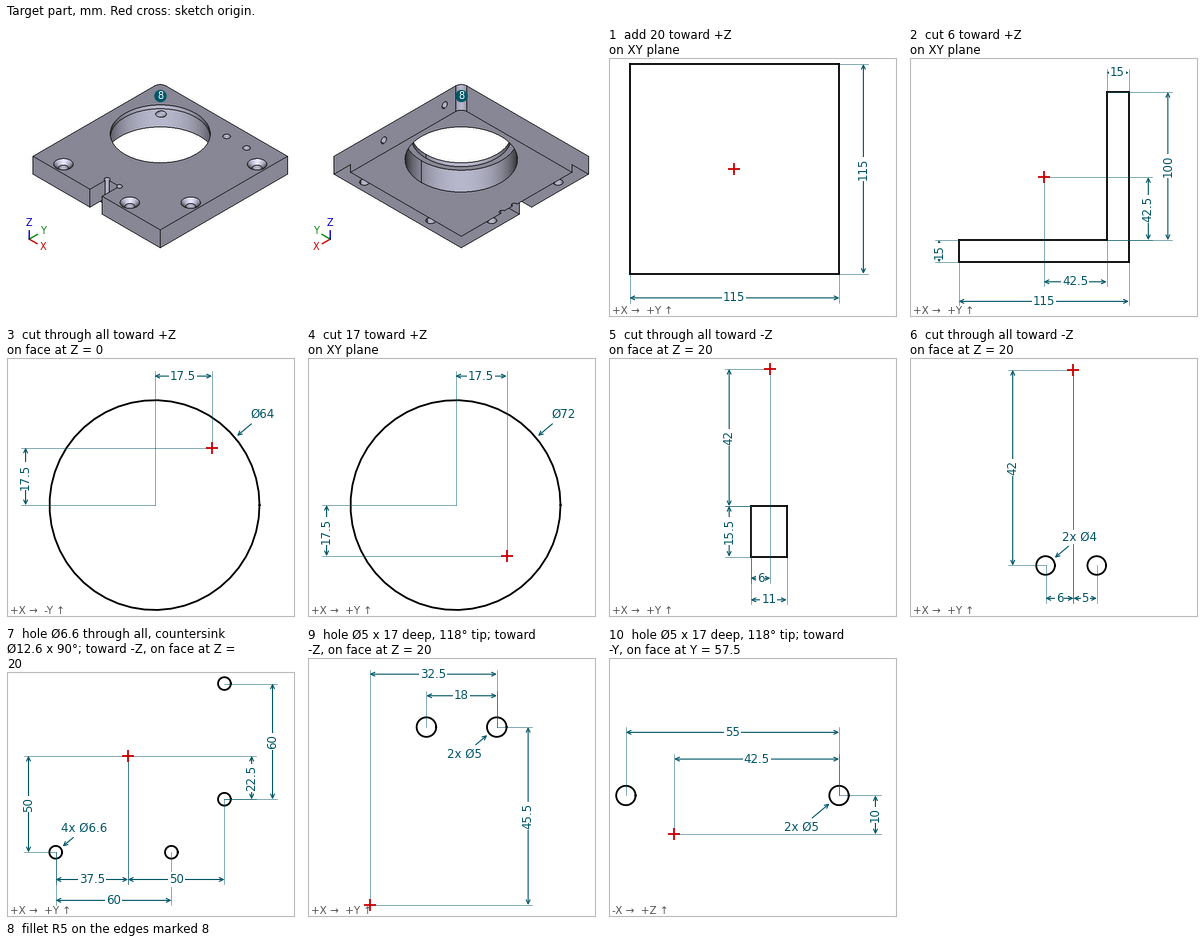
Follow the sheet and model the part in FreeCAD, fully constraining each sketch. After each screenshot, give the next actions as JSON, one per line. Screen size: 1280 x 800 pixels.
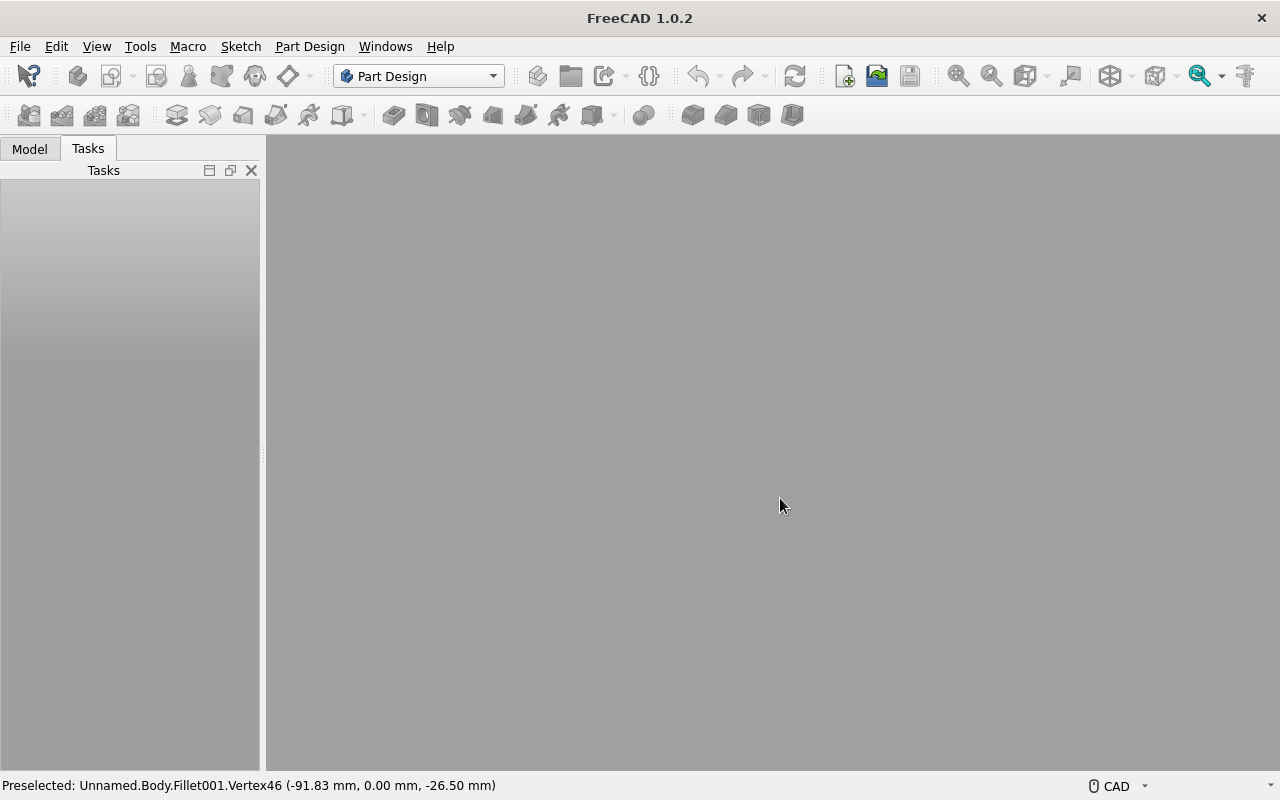
{"action": "key", "text": "ctrl+n"}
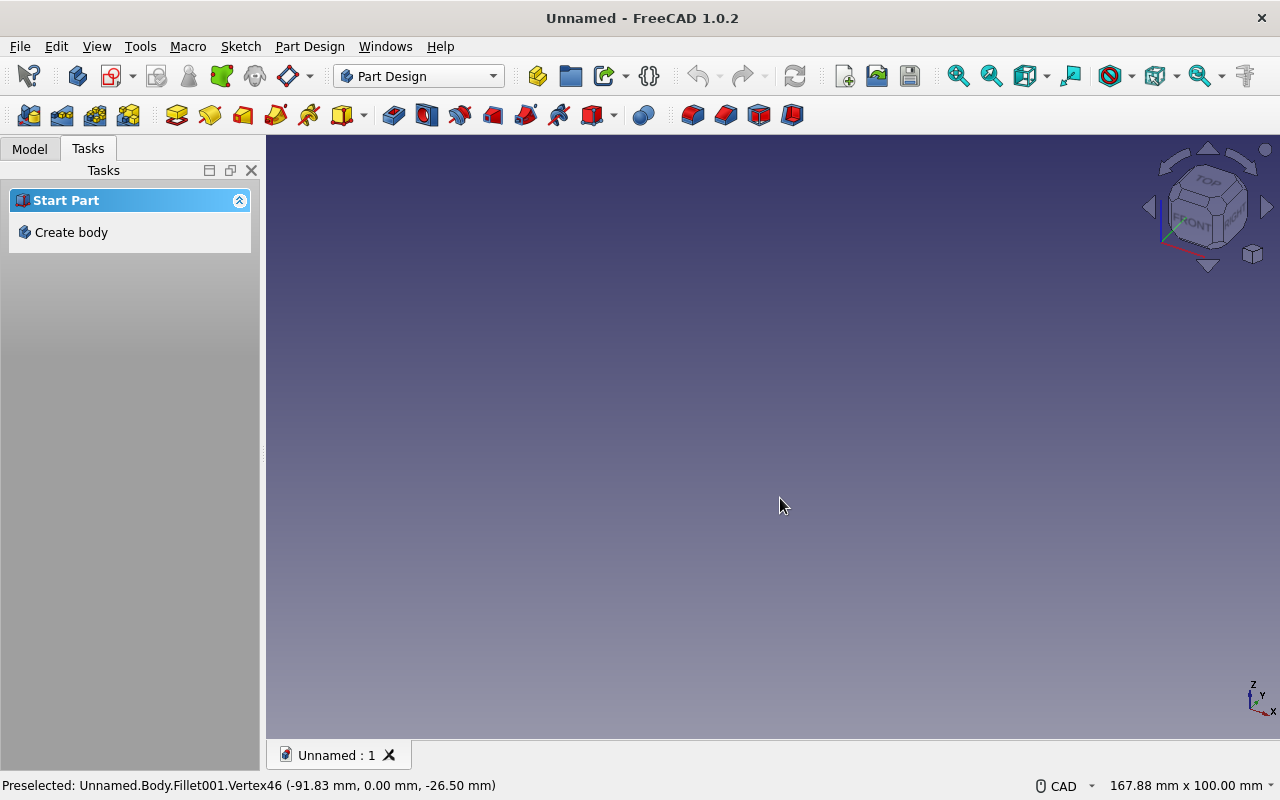
{"action": "left_click", "coordinate": [110, 76]}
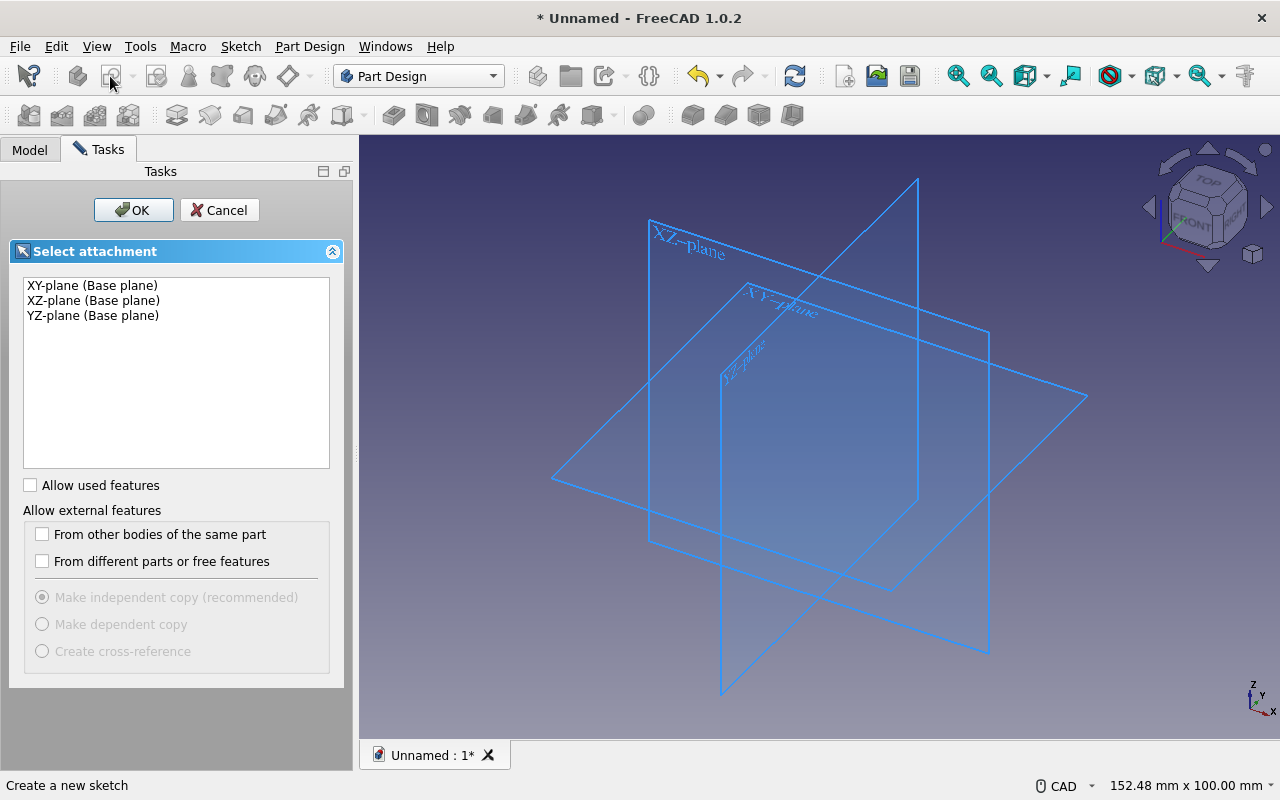
{"action": "left_click", "coordinate": [84, 286]}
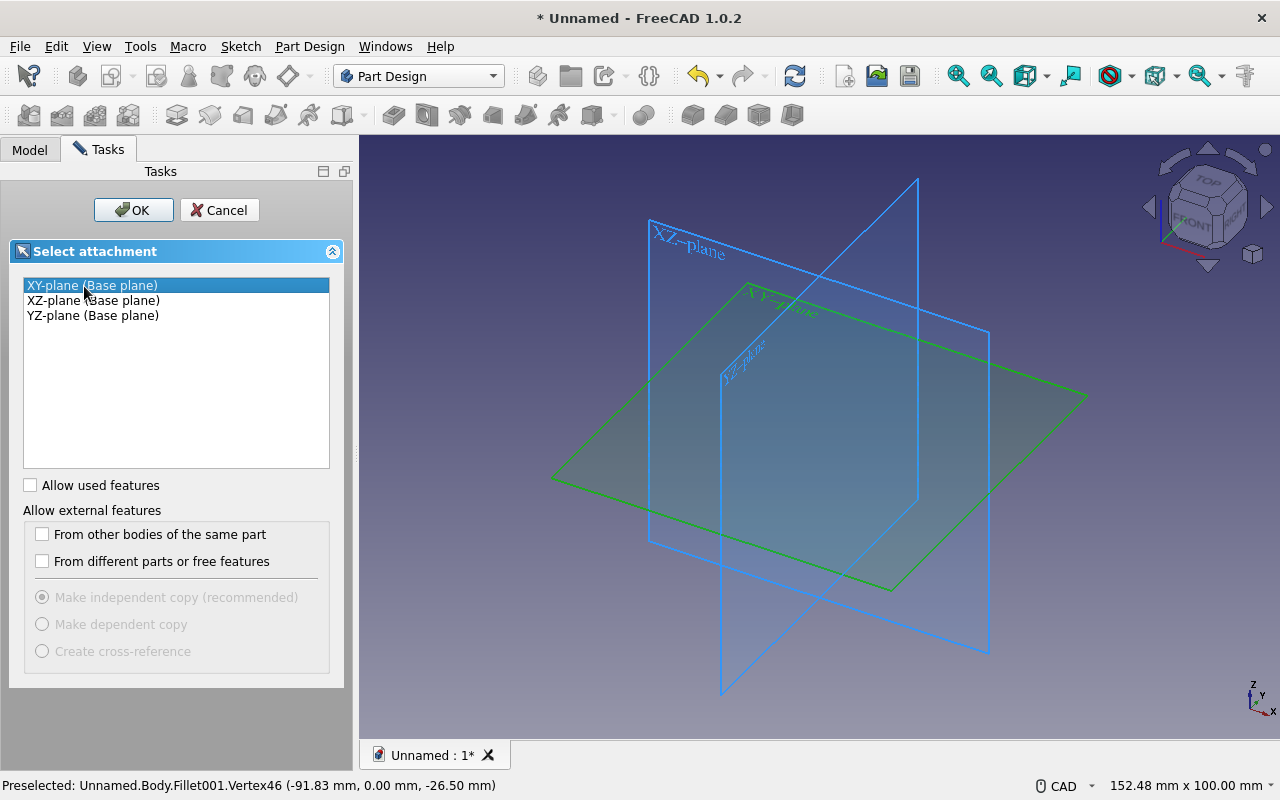
{"action": "left_click", "coordinate": [134, 210]}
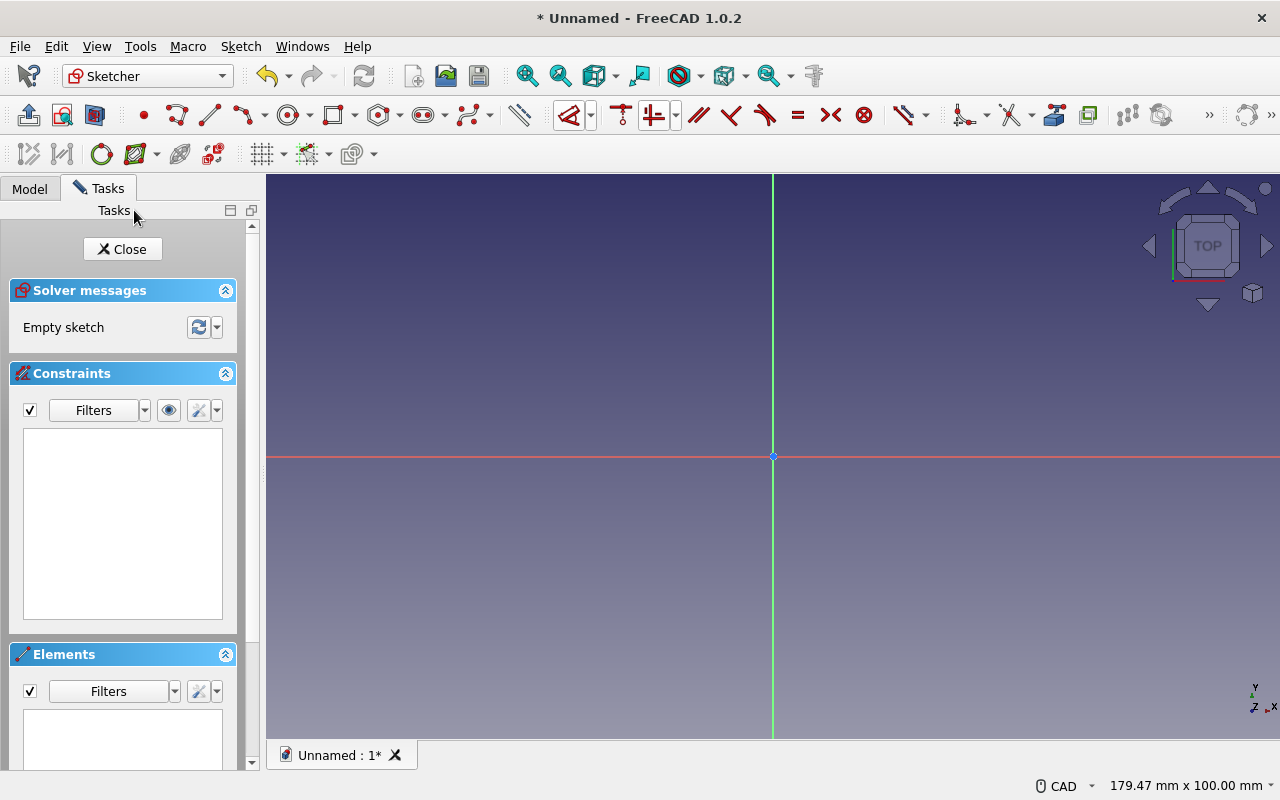
{"action": "scroll", "coordinate": [621, 456], "scroll_direction": "down", "scroll_amount": 3}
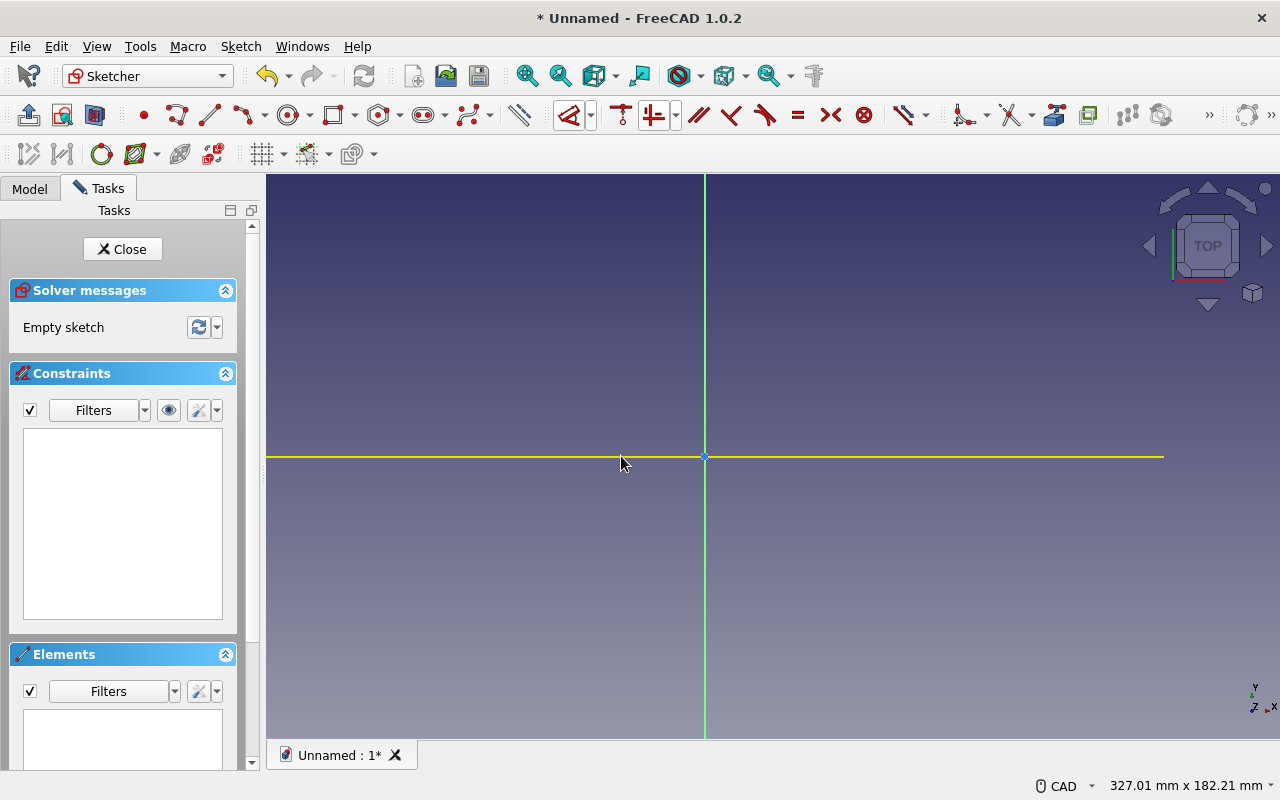
{"action": "key", "text": "g v"}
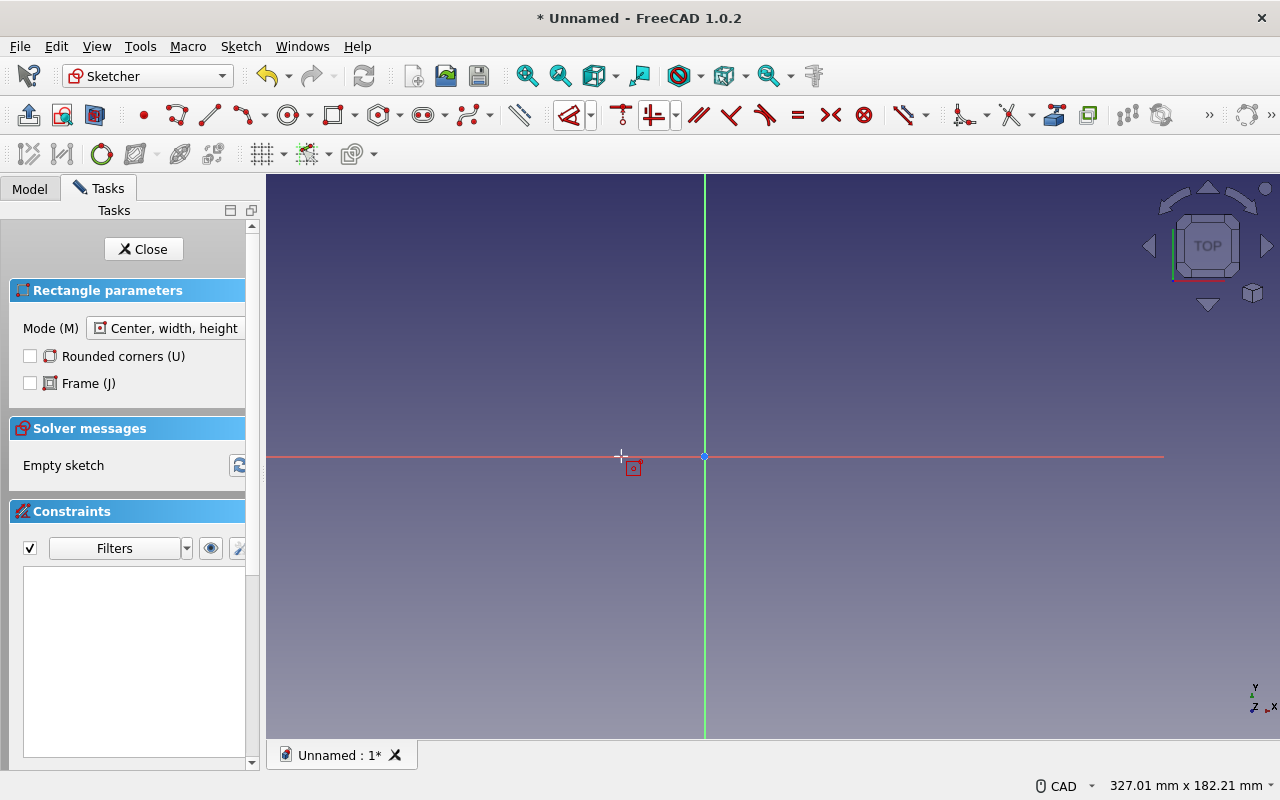
{"action": "left_click", "coordinate": [705, 456]}
{"action": "left_click", "coordinate": [883, 278]}
{"action": "key", "text": "Escape"}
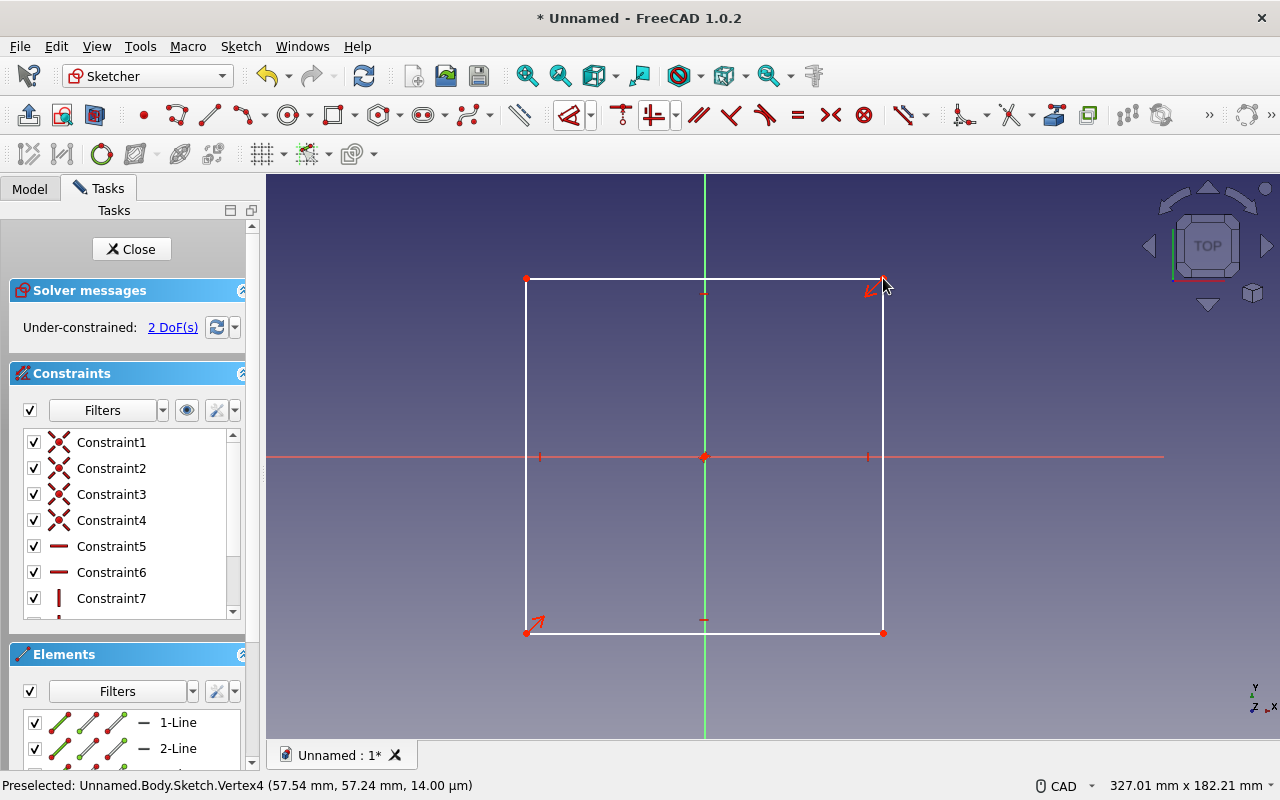
{"action": "left_click", "coordinate": [633, 634]}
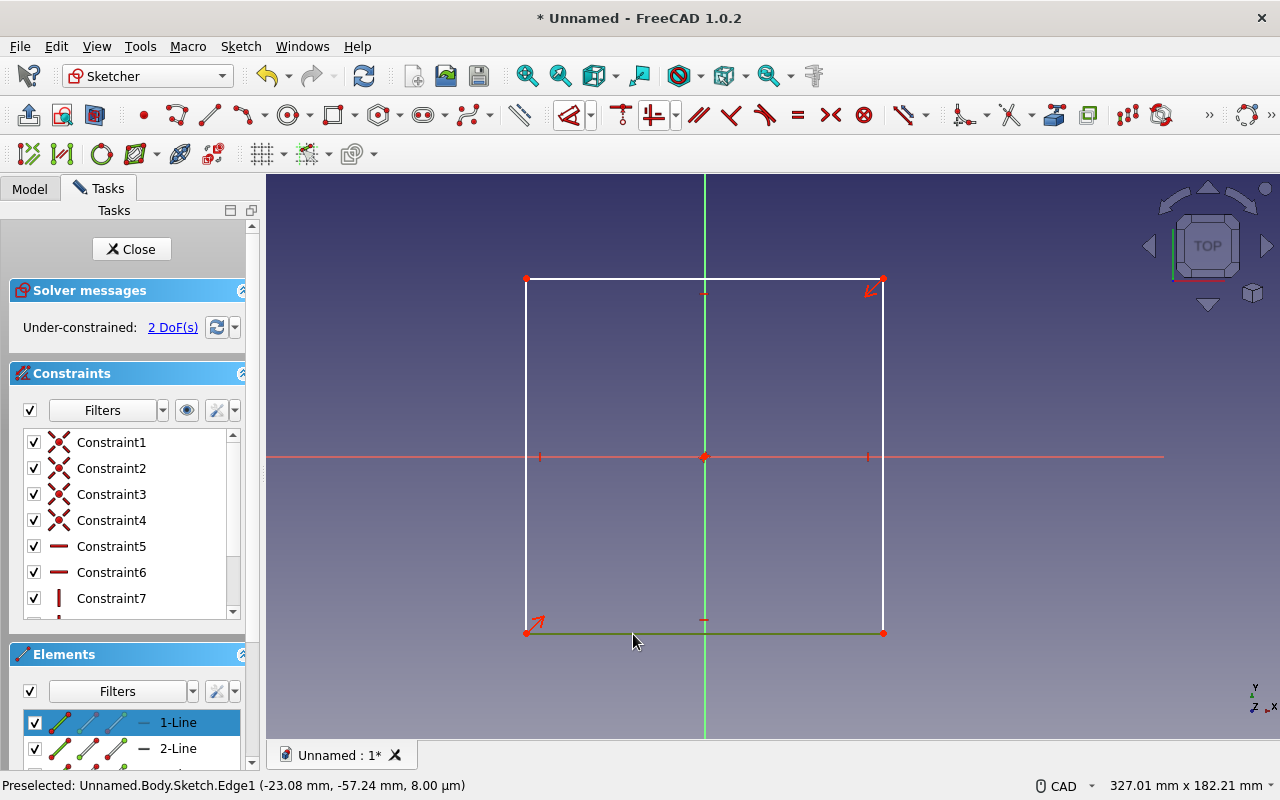
{"action": "left_click", "coordinate": [590, 116]}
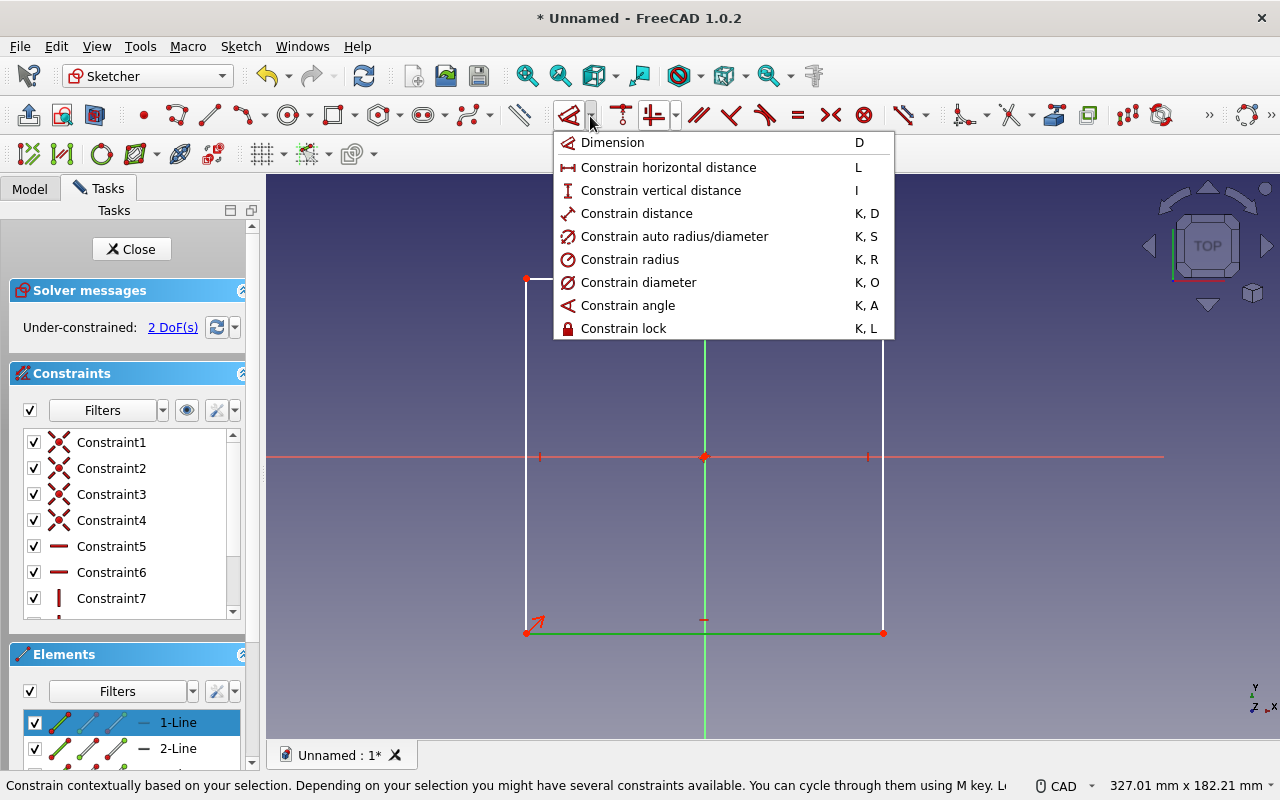
{"action": "left_click", "coordinate": [724, 168]}